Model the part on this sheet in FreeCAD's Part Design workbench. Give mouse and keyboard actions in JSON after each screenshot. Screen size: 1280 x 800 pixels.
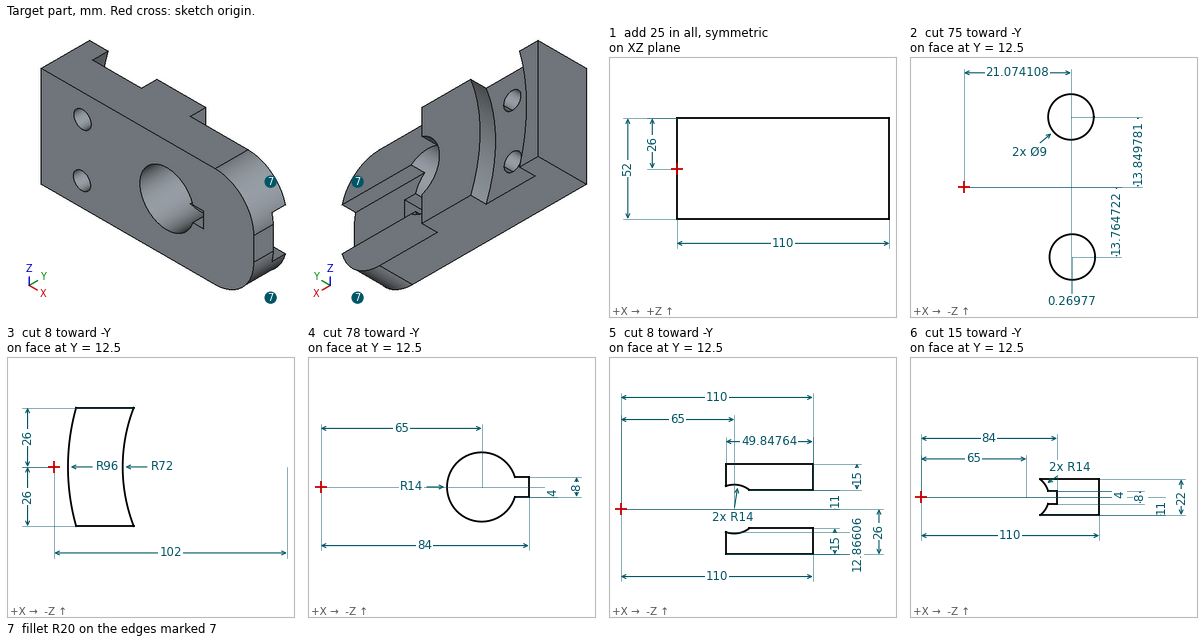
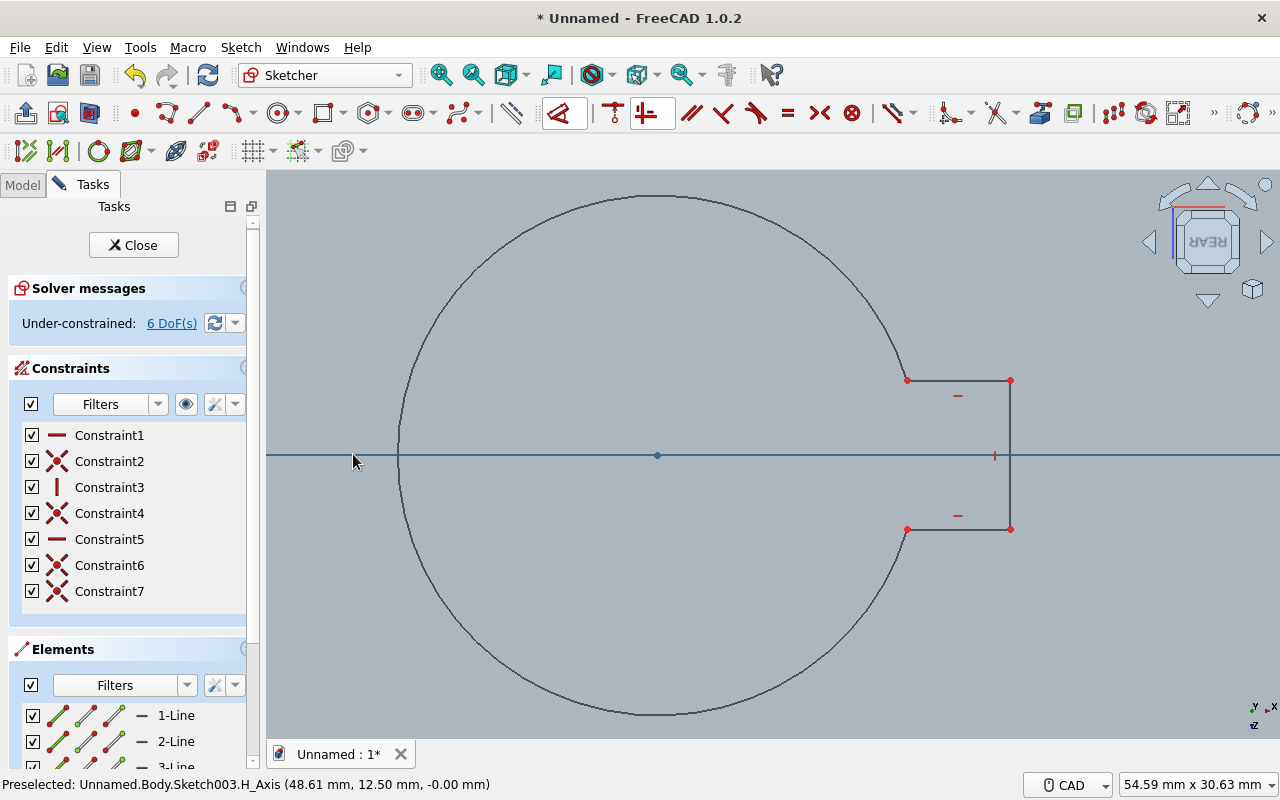
{"action": "left_click", "coordinate": [614, 114]}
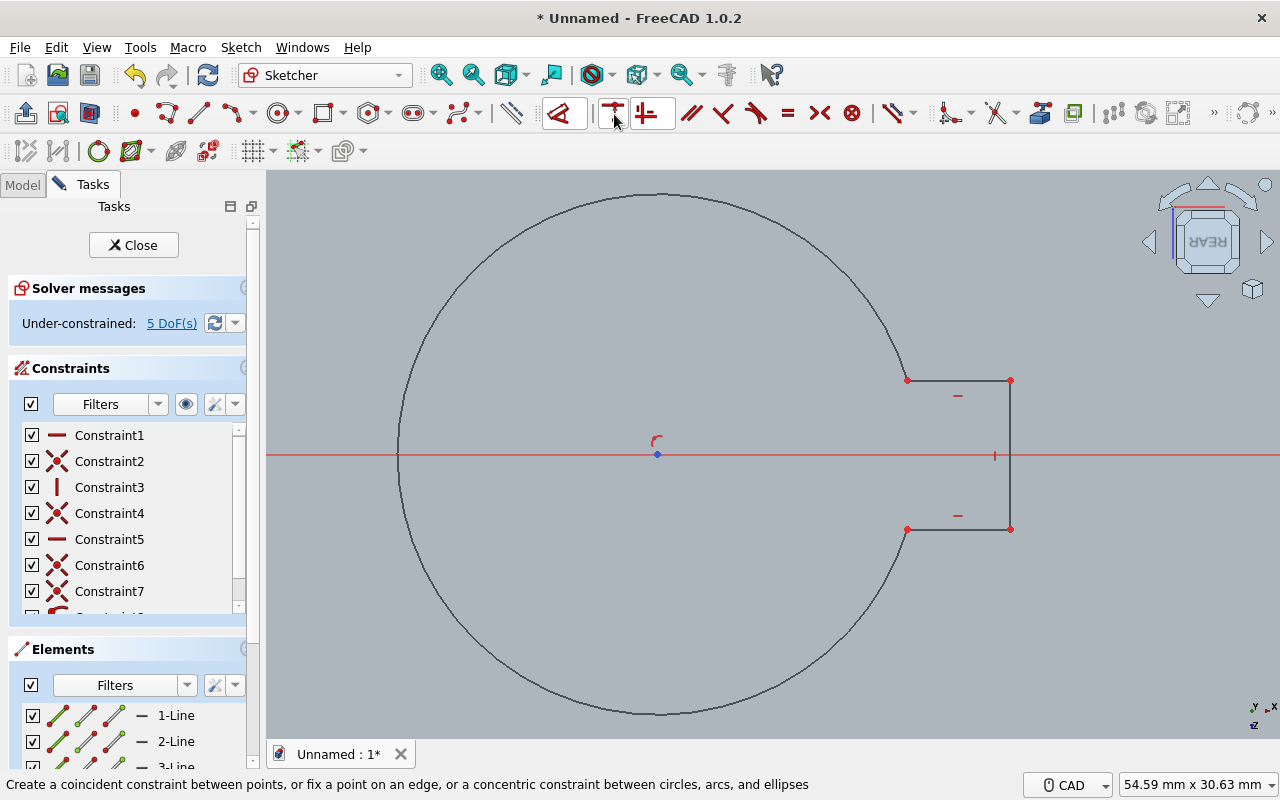
{"action": "left_click", "coordinate": [550, 217]}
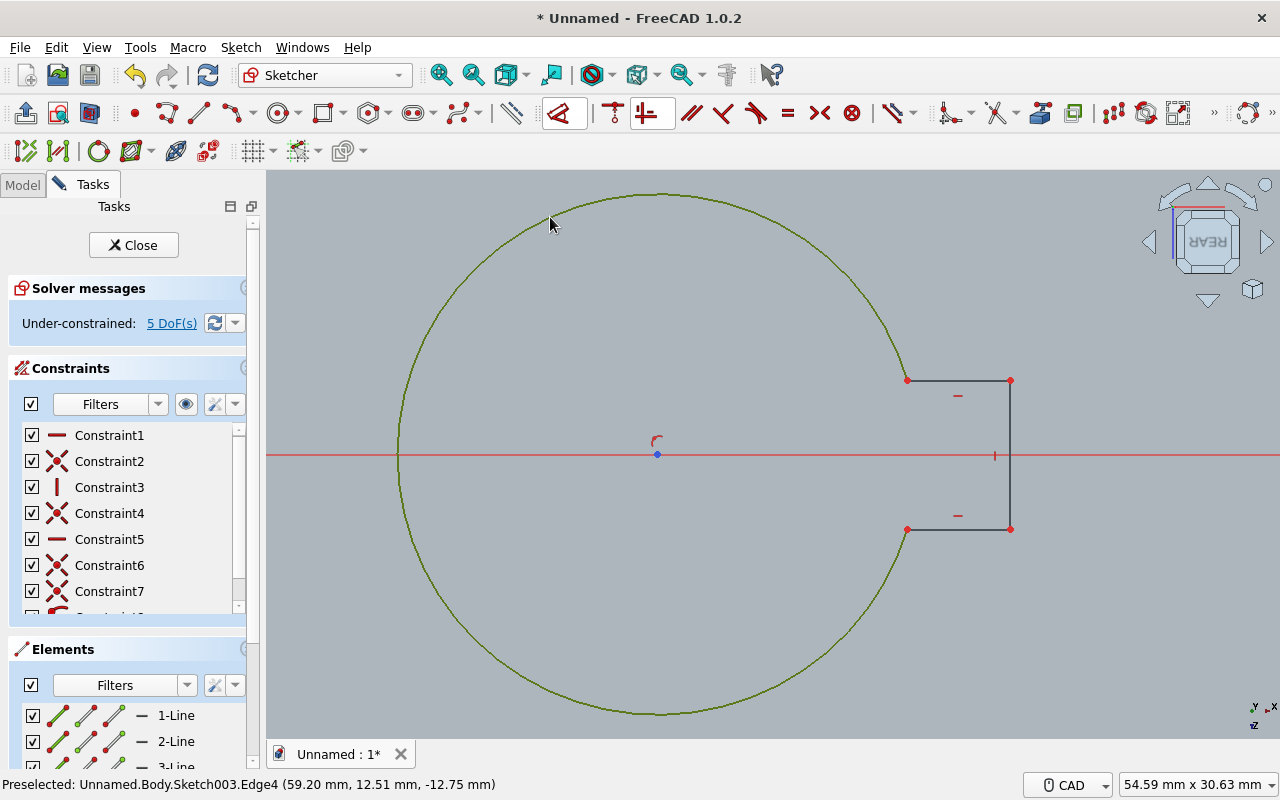
{"action": "left_click", "coordinate": [582, 114]}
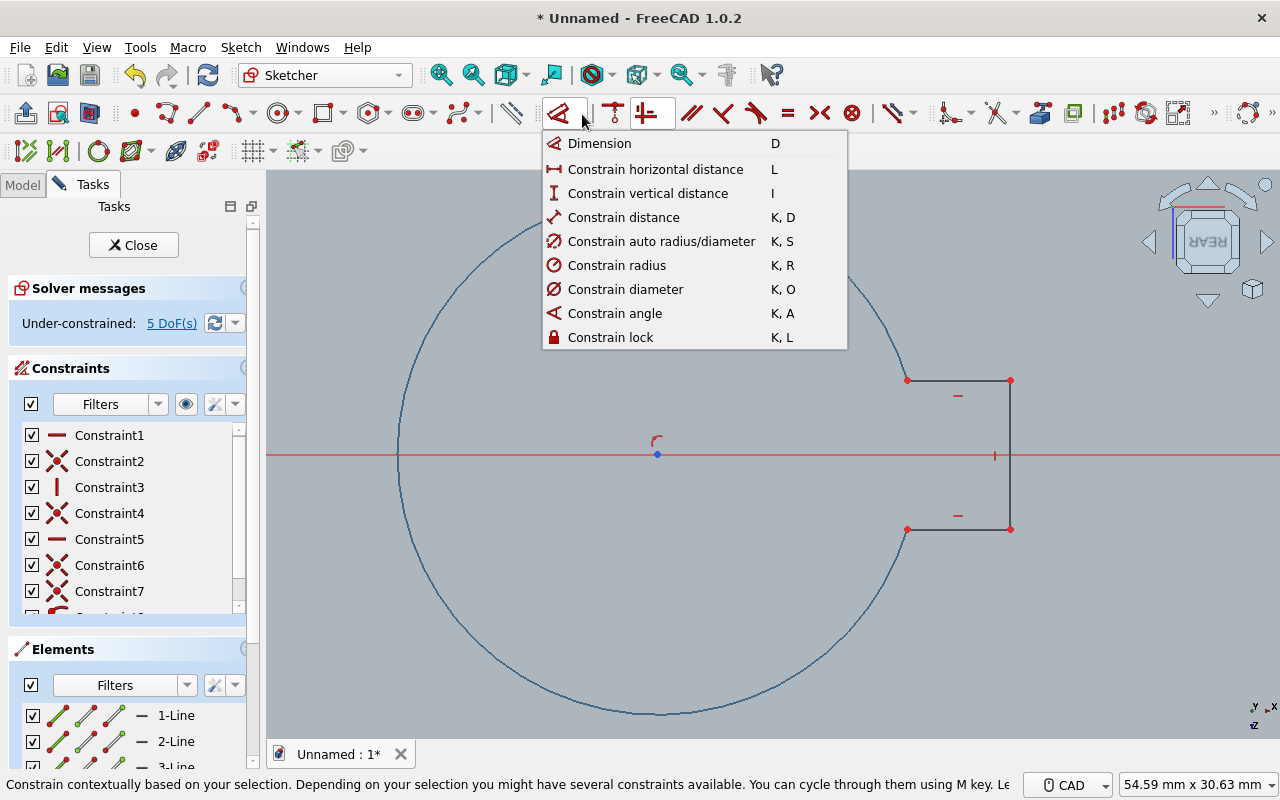
{"action": "left_click", "coordinate": [695, 265]}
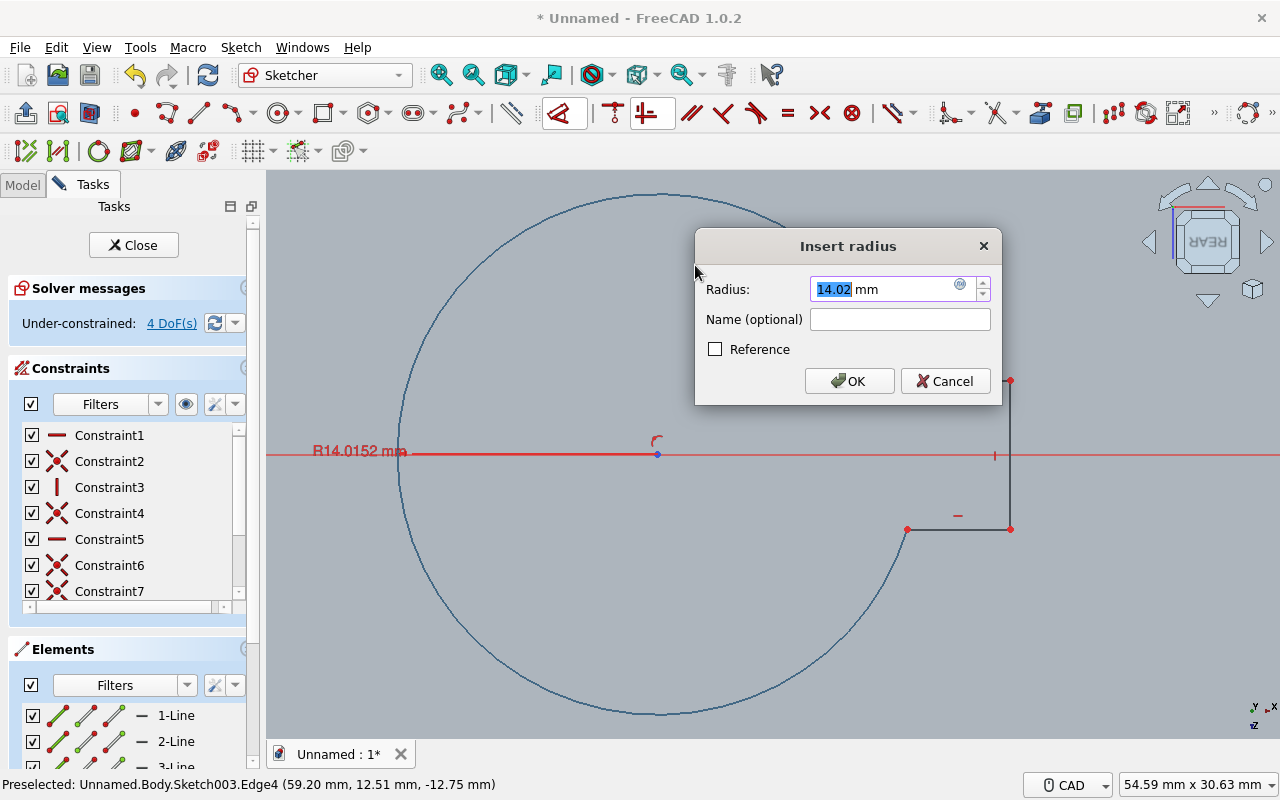
{"action": "type", "text": "14"}
{"action": "key", "text": "Return"}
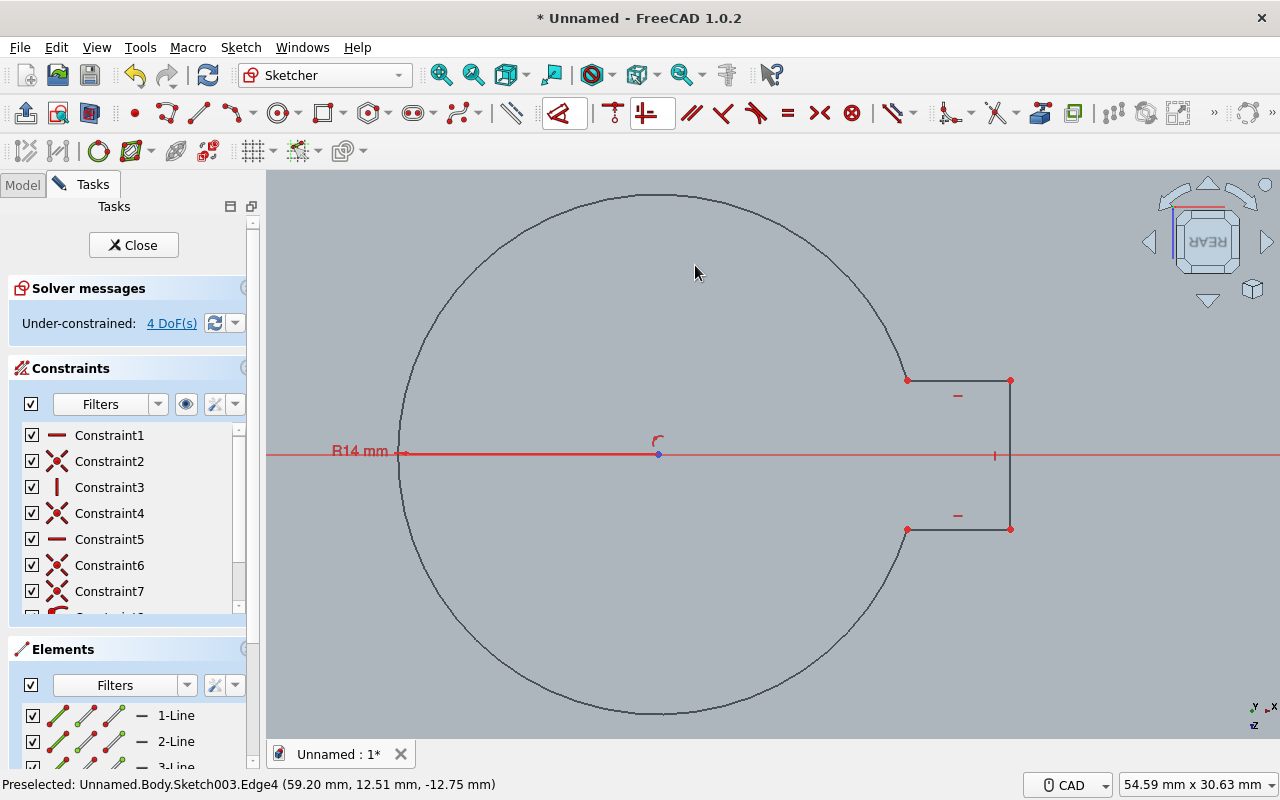
{"action": "left_click", "coordinate": [1010, 485]}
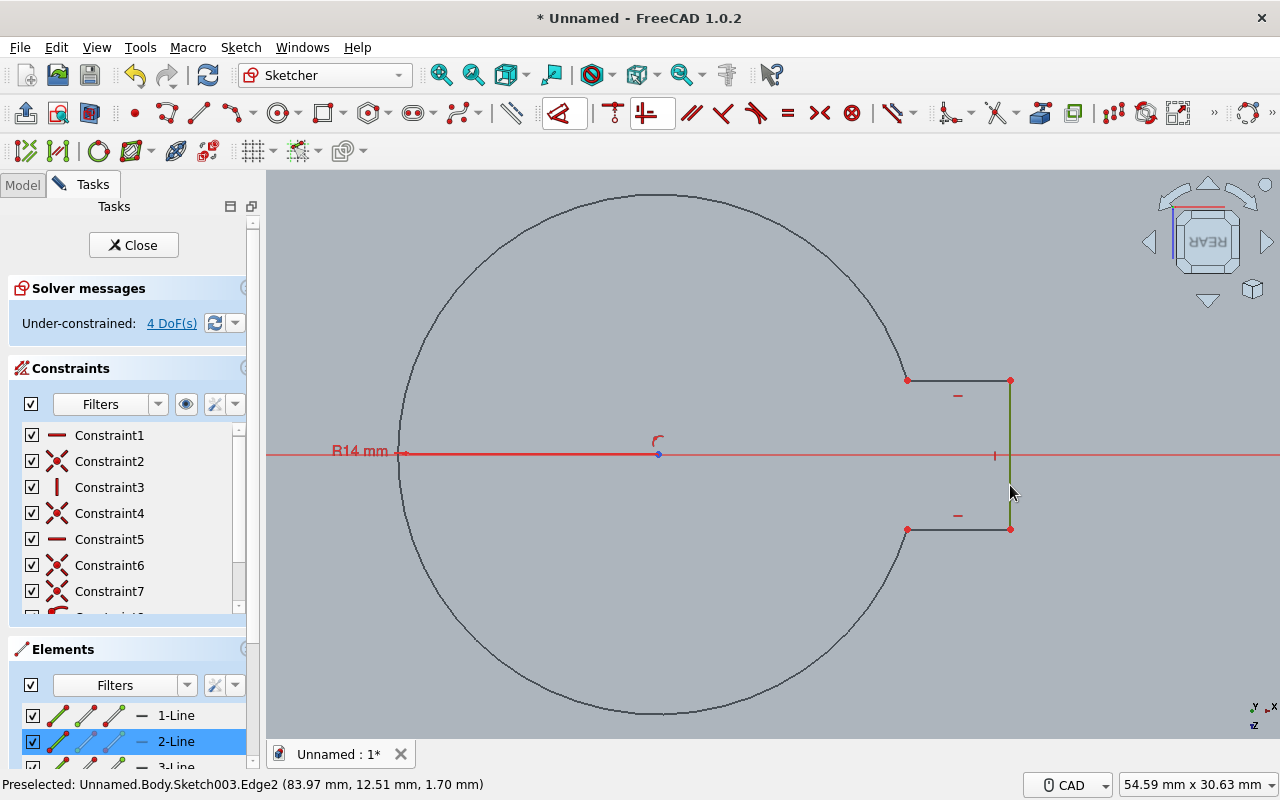
{"action": "left_click", "coordinate": [582, 114]}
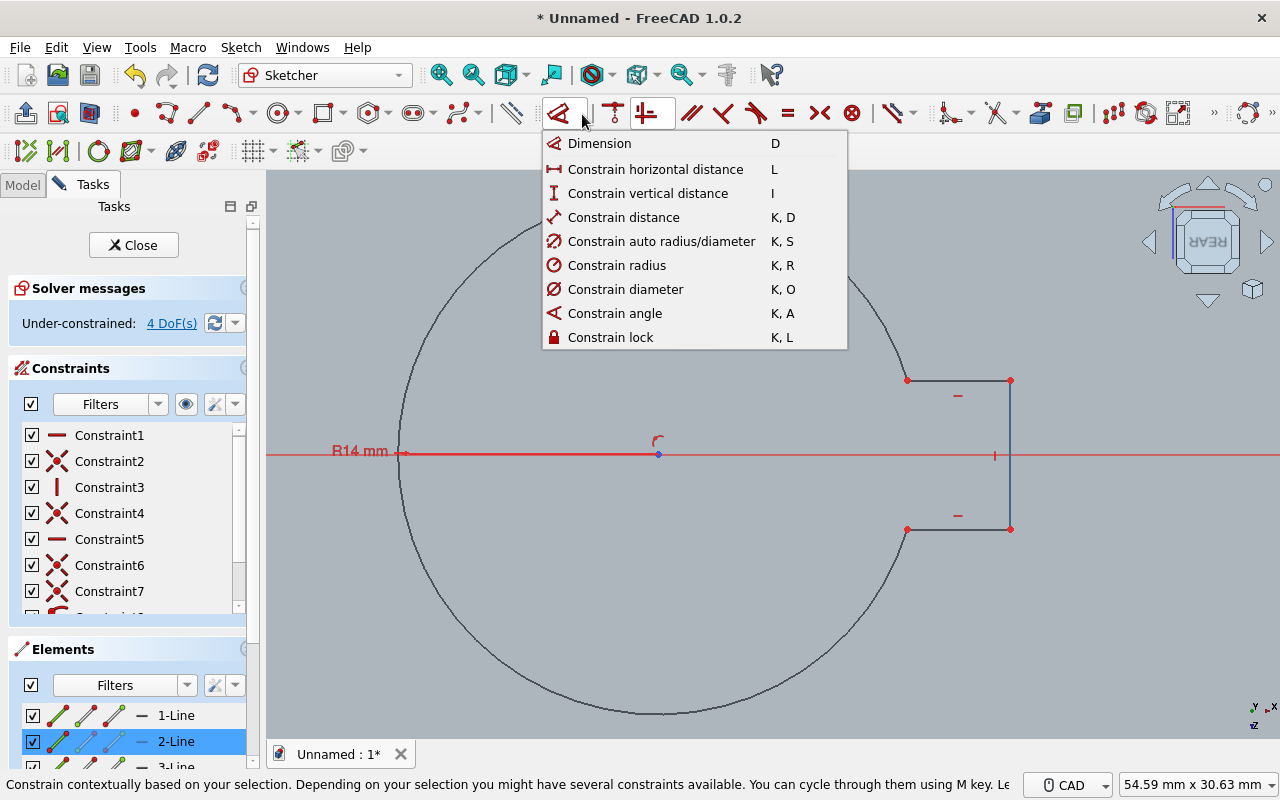
{"action": "left_click", "coordinate": [695, 193]}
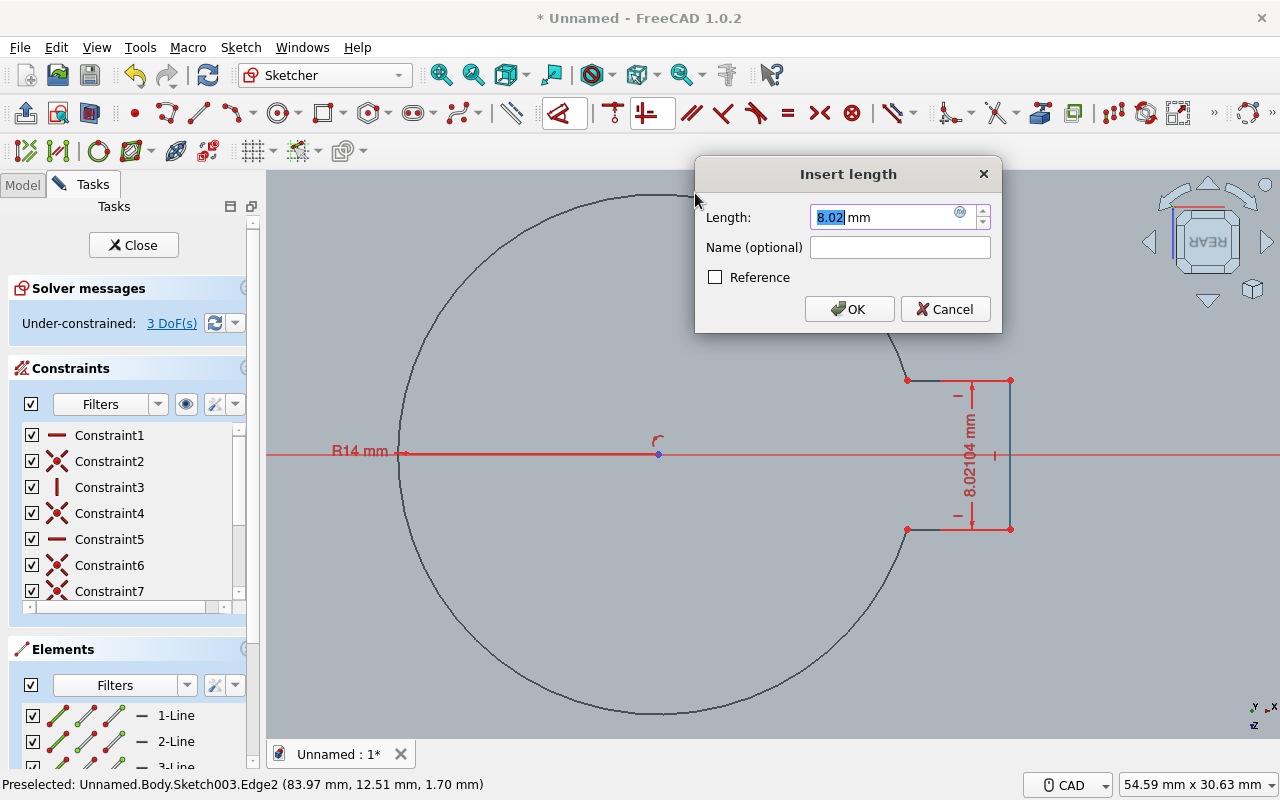
{"action": "type", "text": "8"}
{"action": "key", "text": "Return"}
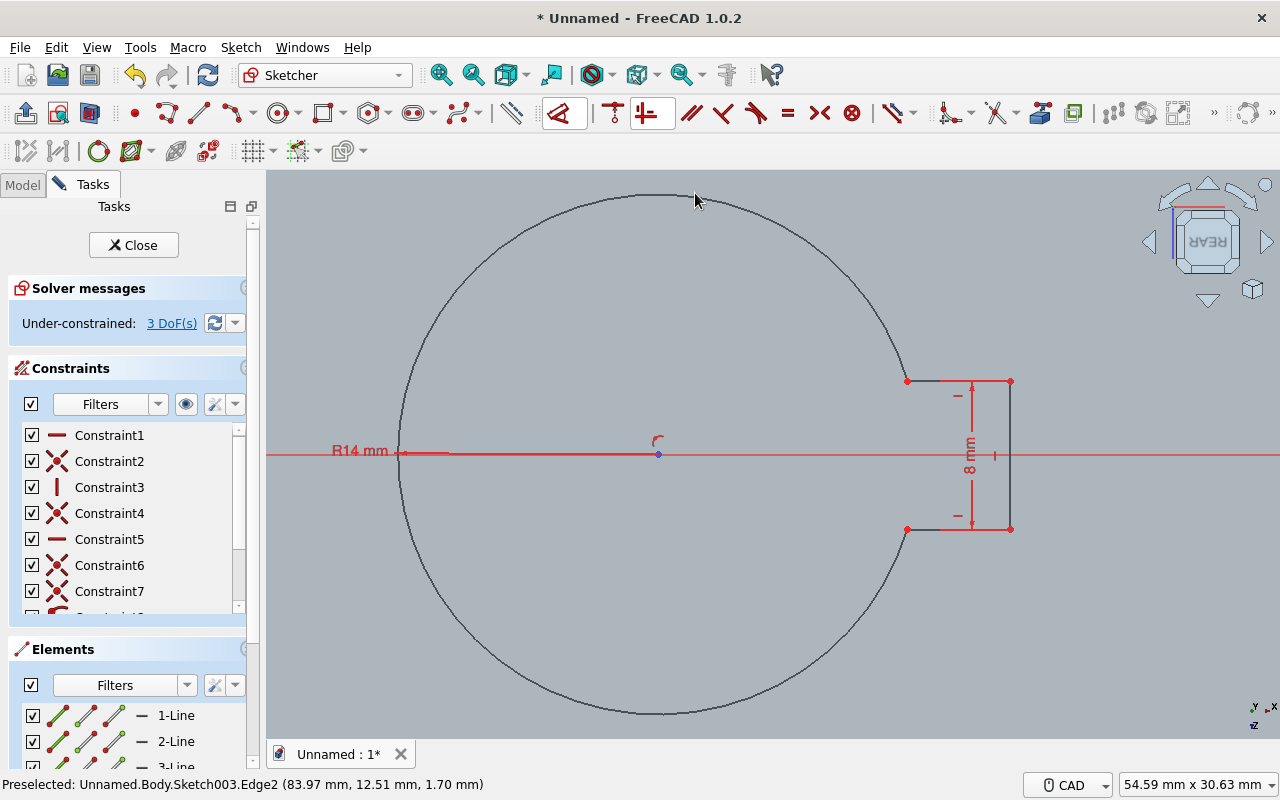
{"action": "left_click", "coordinate": [907, 530]}